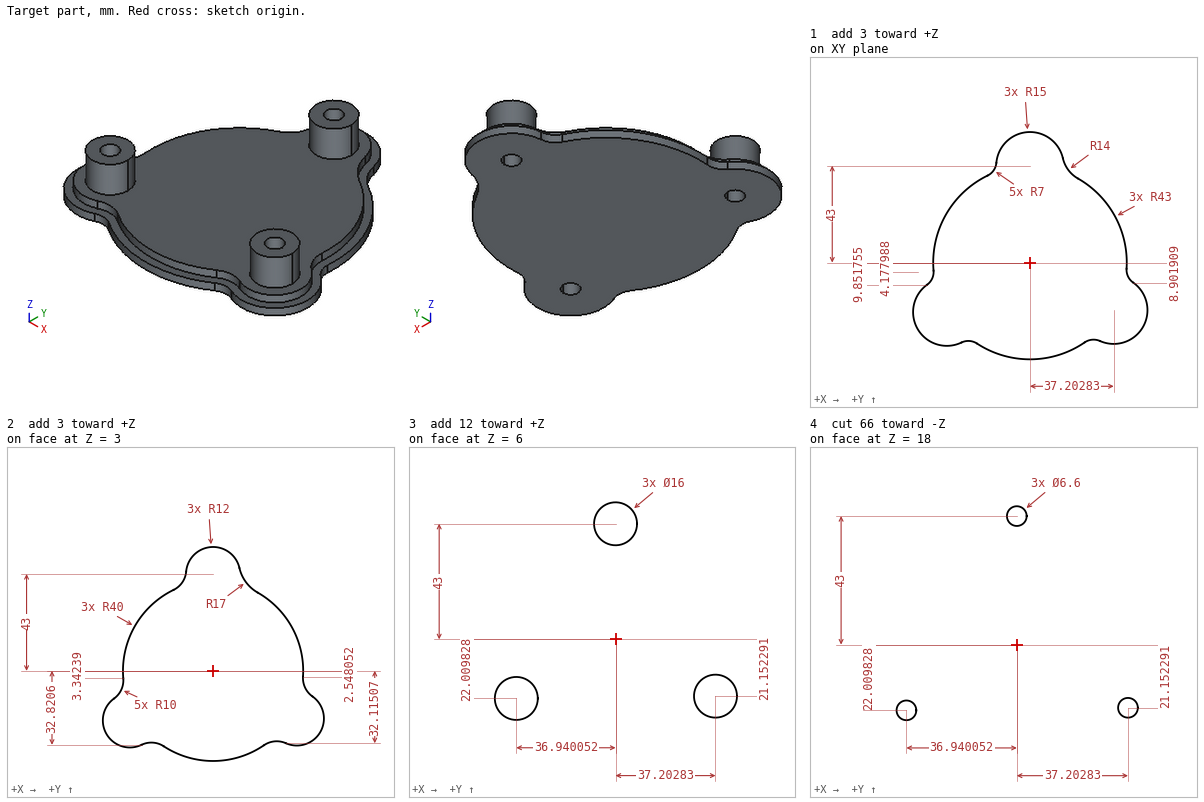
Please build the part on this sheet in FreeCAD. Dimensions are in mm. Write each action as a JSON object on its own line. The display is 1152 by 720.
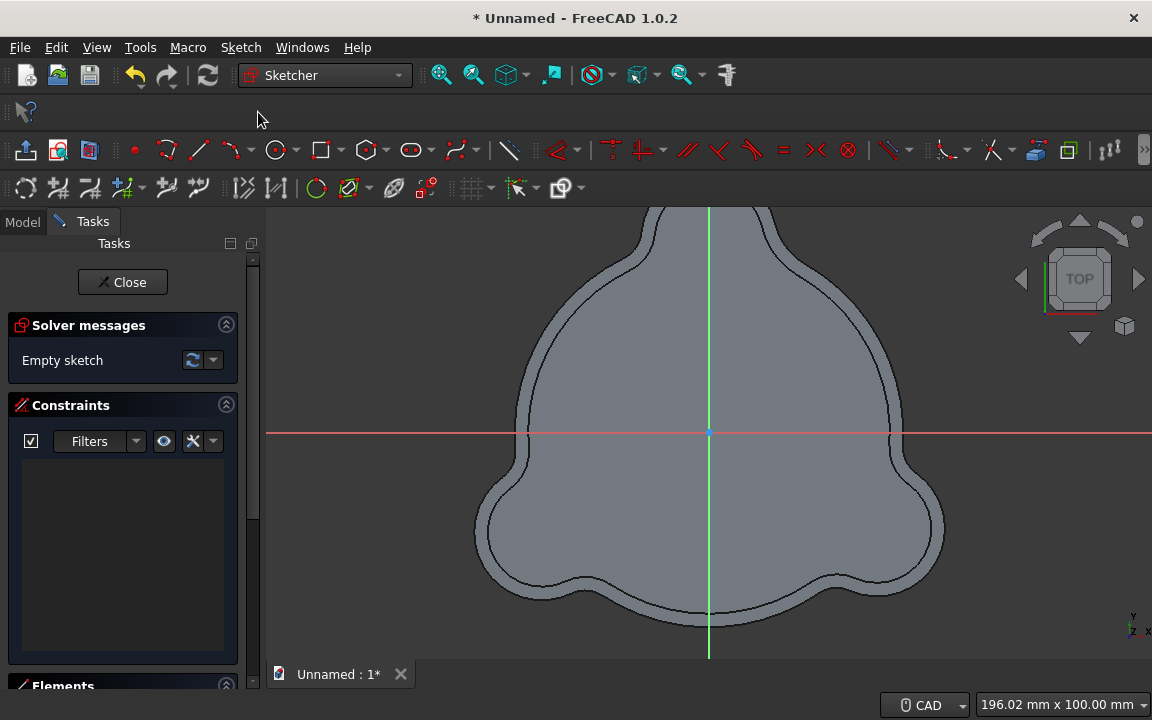
{"action": "scroll", "coordinate": [328, 631], "scroll_direction": "down", "scroll_amount": 1}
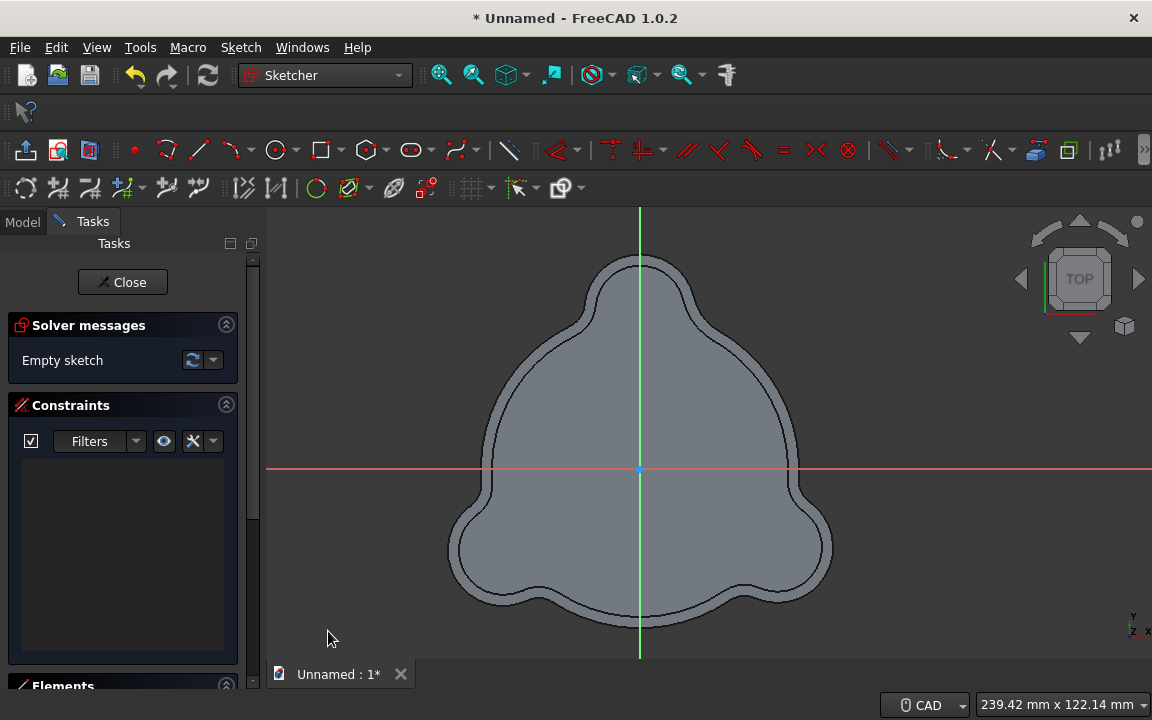
{"action": "left_click", "coordinate": [276, 150]}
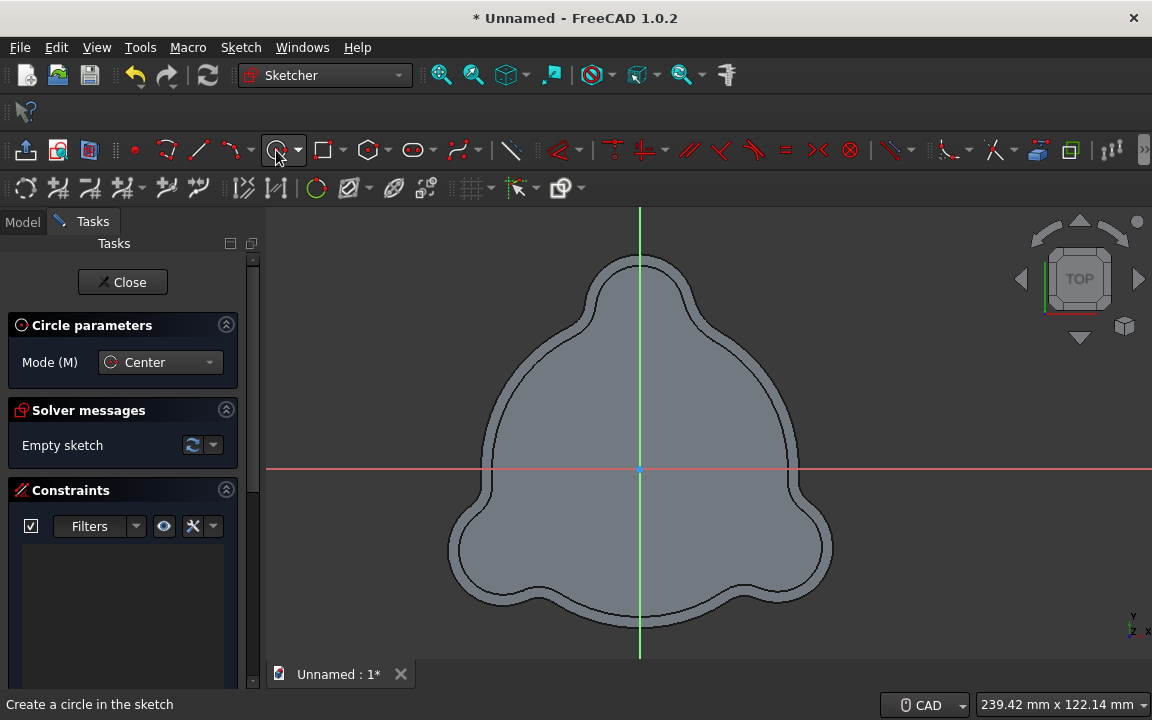
{"action": "left_click", "coordinate": [640, 310]}
{"action": "left_click", "coordinate": [661, 289]}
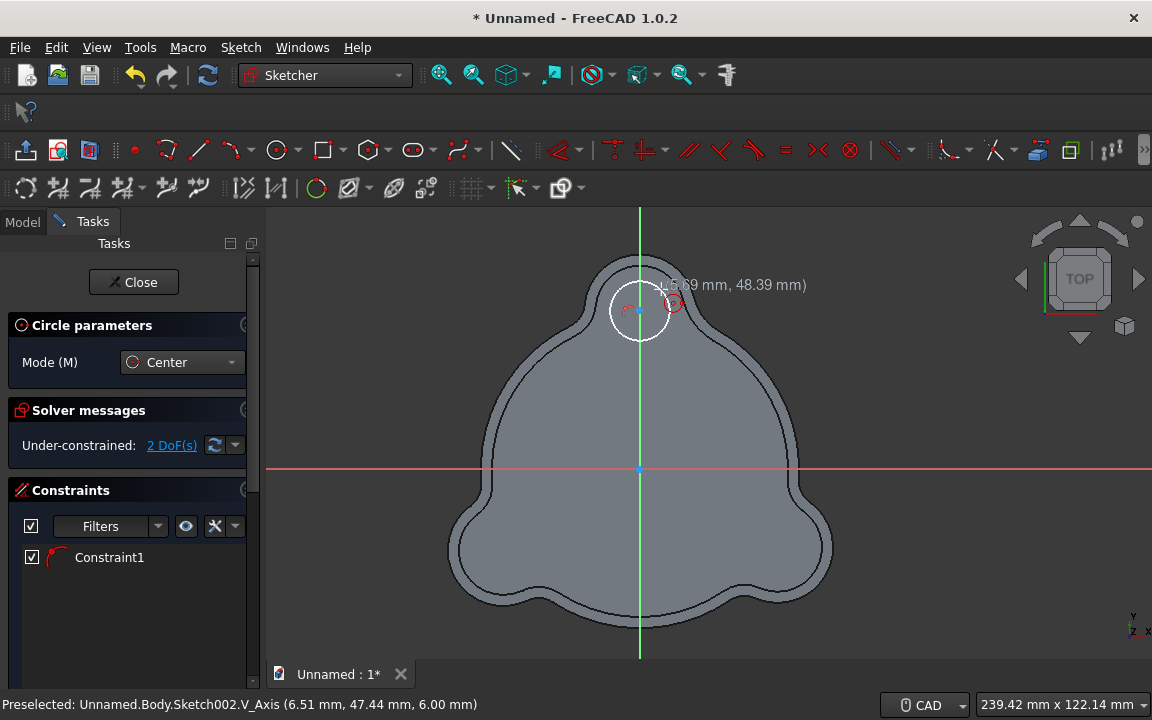
{"action": "left_click", "coordinate": [778, 547]}
{"action": "left_click", "coordinate": [799, 526]}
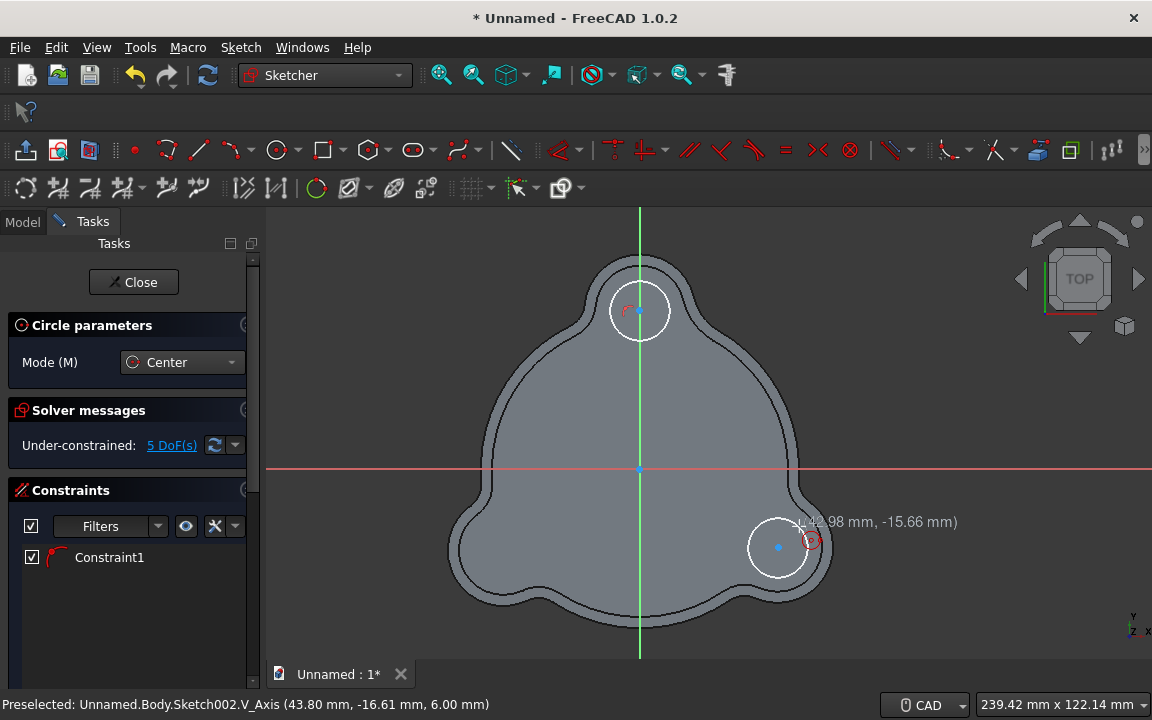
{"action": "left_click", "coordinate": [503, 551]}
{"action": "left_click", "coordinate": [524, 530]}
{"action": "key", "text": "Escape"}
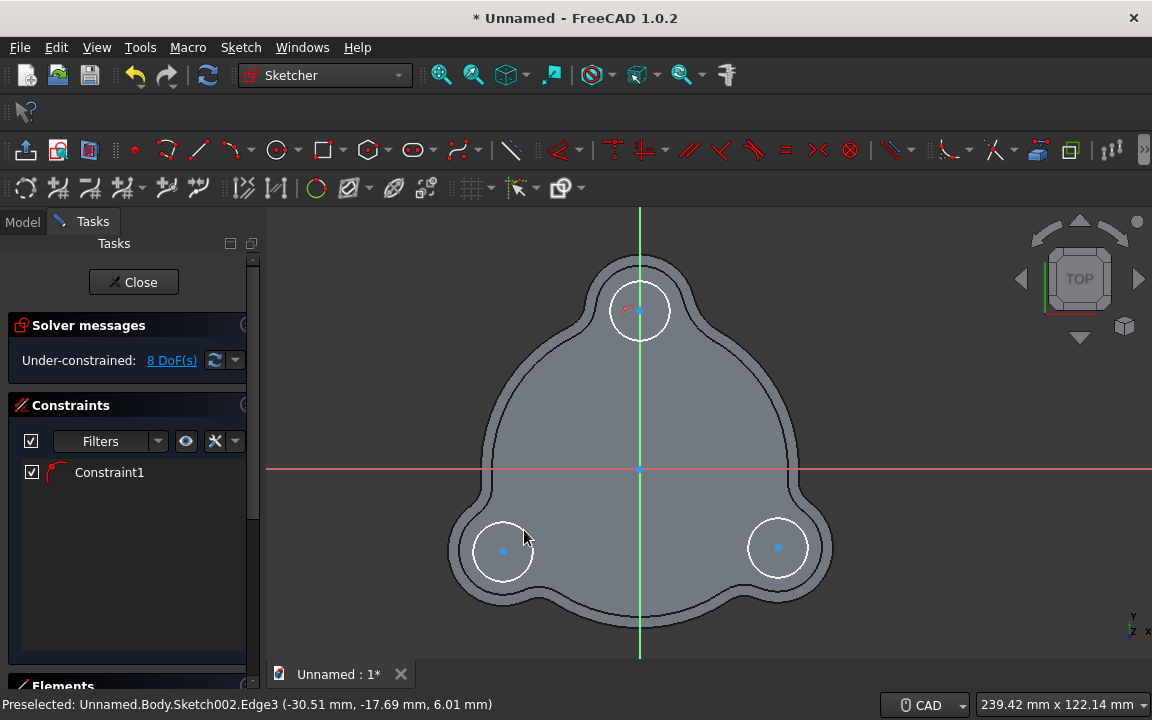
{"action": "left_click", "coordinate": [661, 290]}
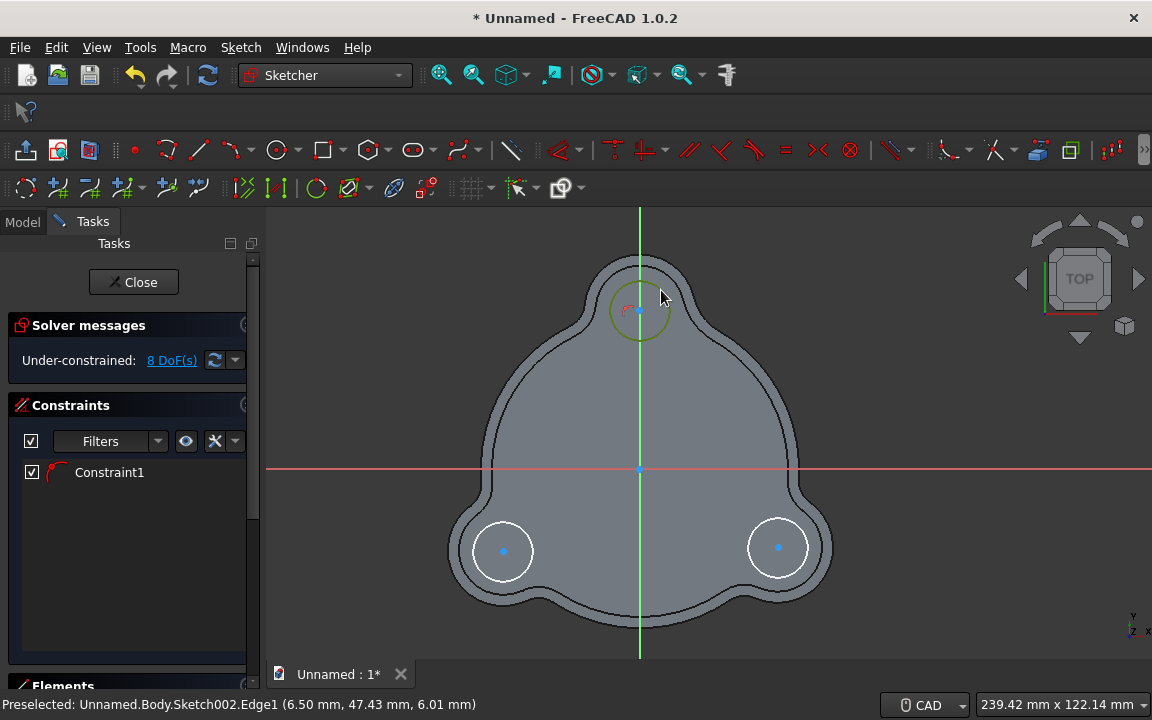
{"action": "left_click", "coordinate": [799, 527]}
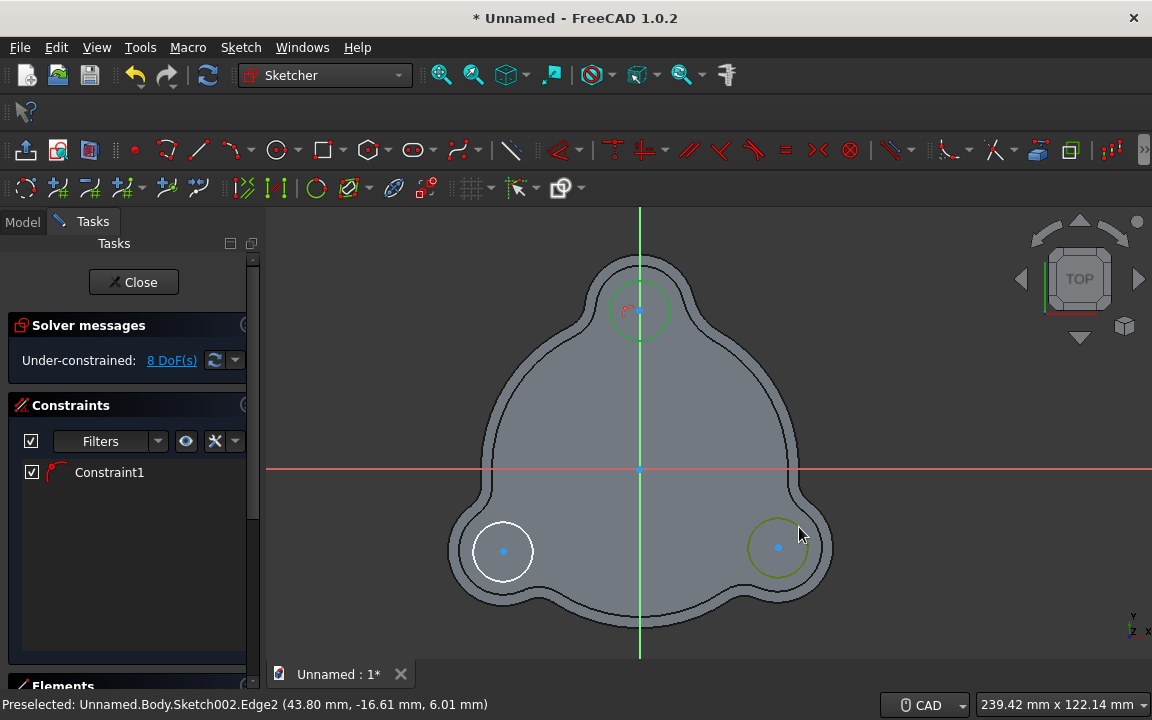
{"action": "left_click", "coordinate": [524, 531]}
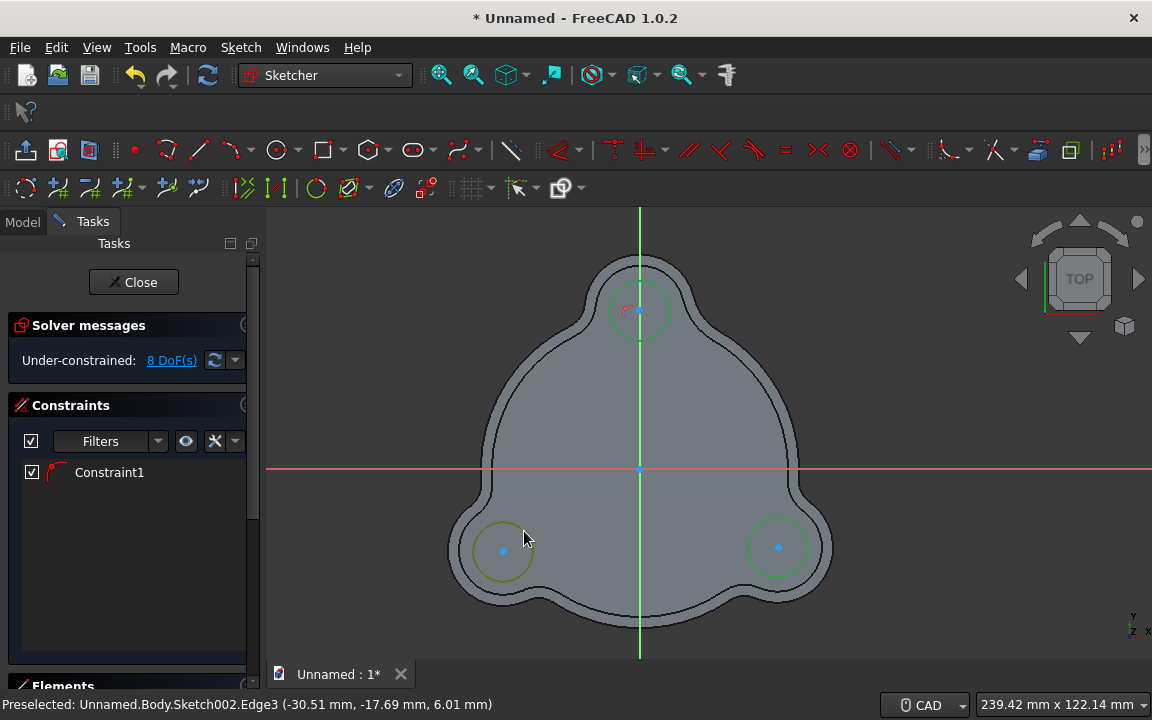
{"action": "left_click", "coordinate": [786, 150]}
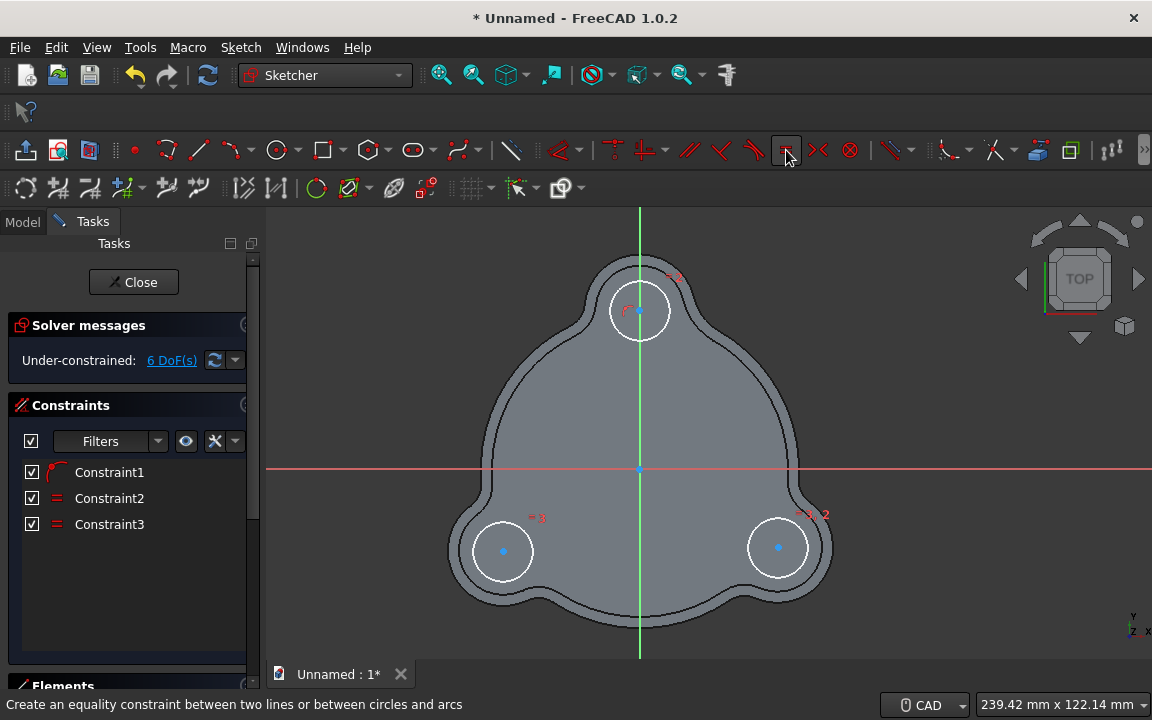
{"action": "key", "text": "d"}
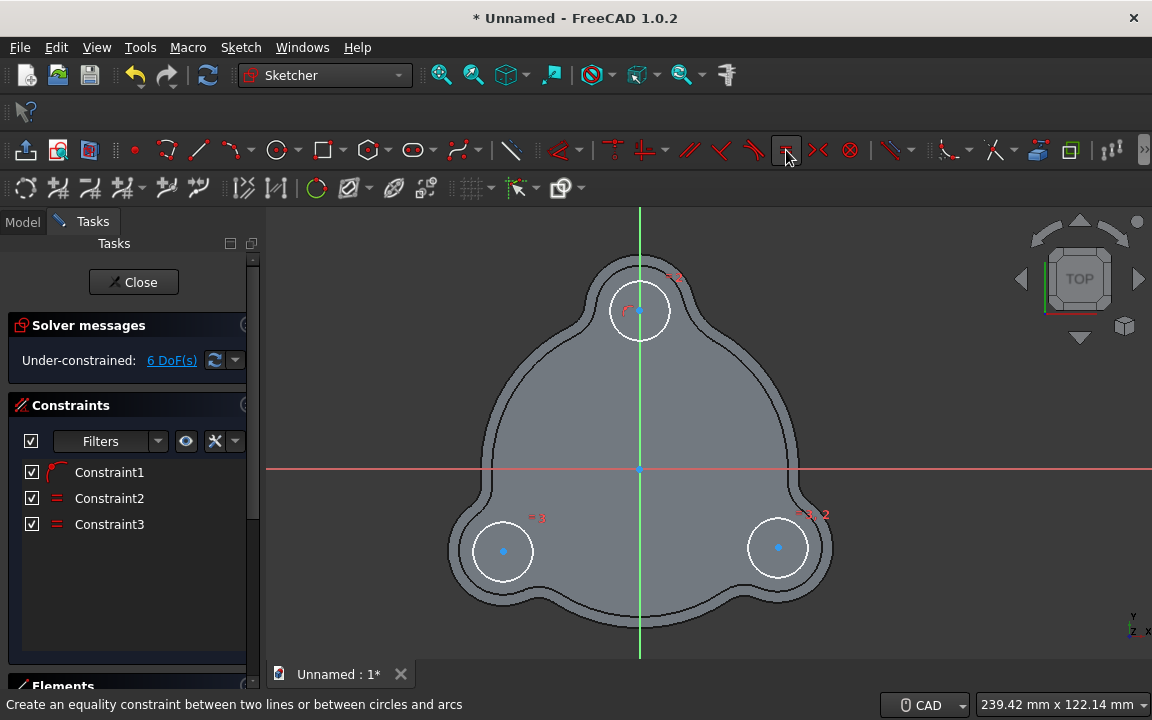
{"action": "left_click", "coordinate": [661, 290]}
{"action": "left_click", "coordinate": [684, 267]}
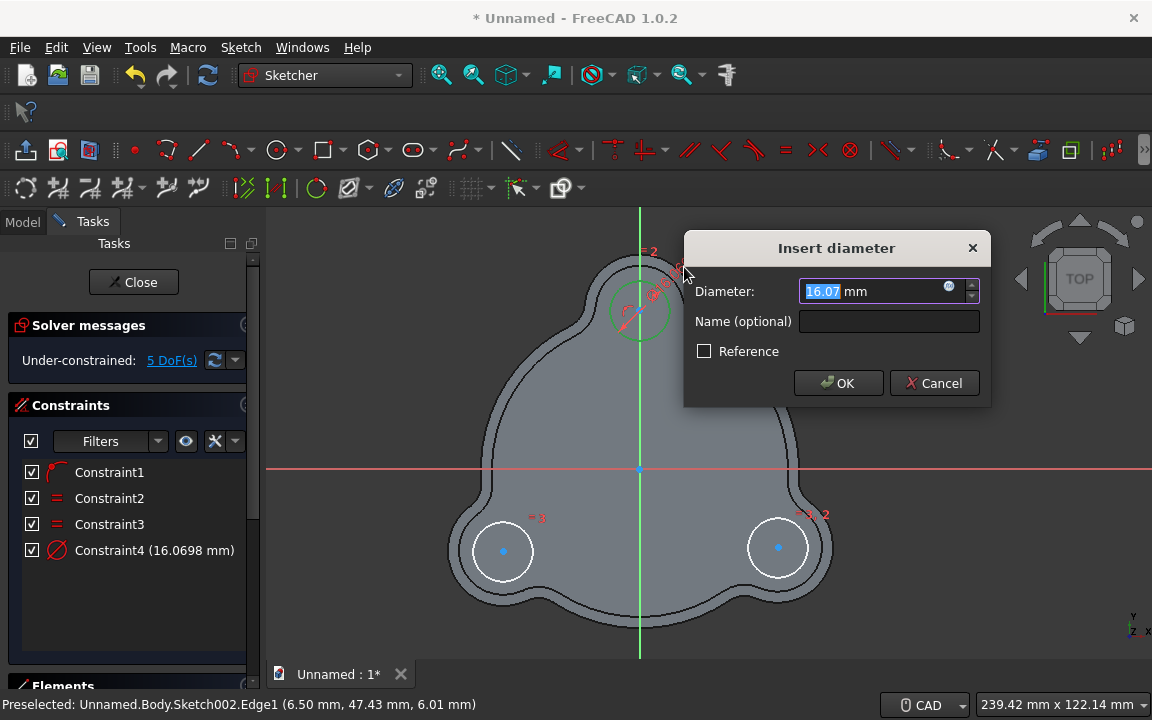
{"action": "type", "text": "16"}
{"action": "key", "text": "Return"}